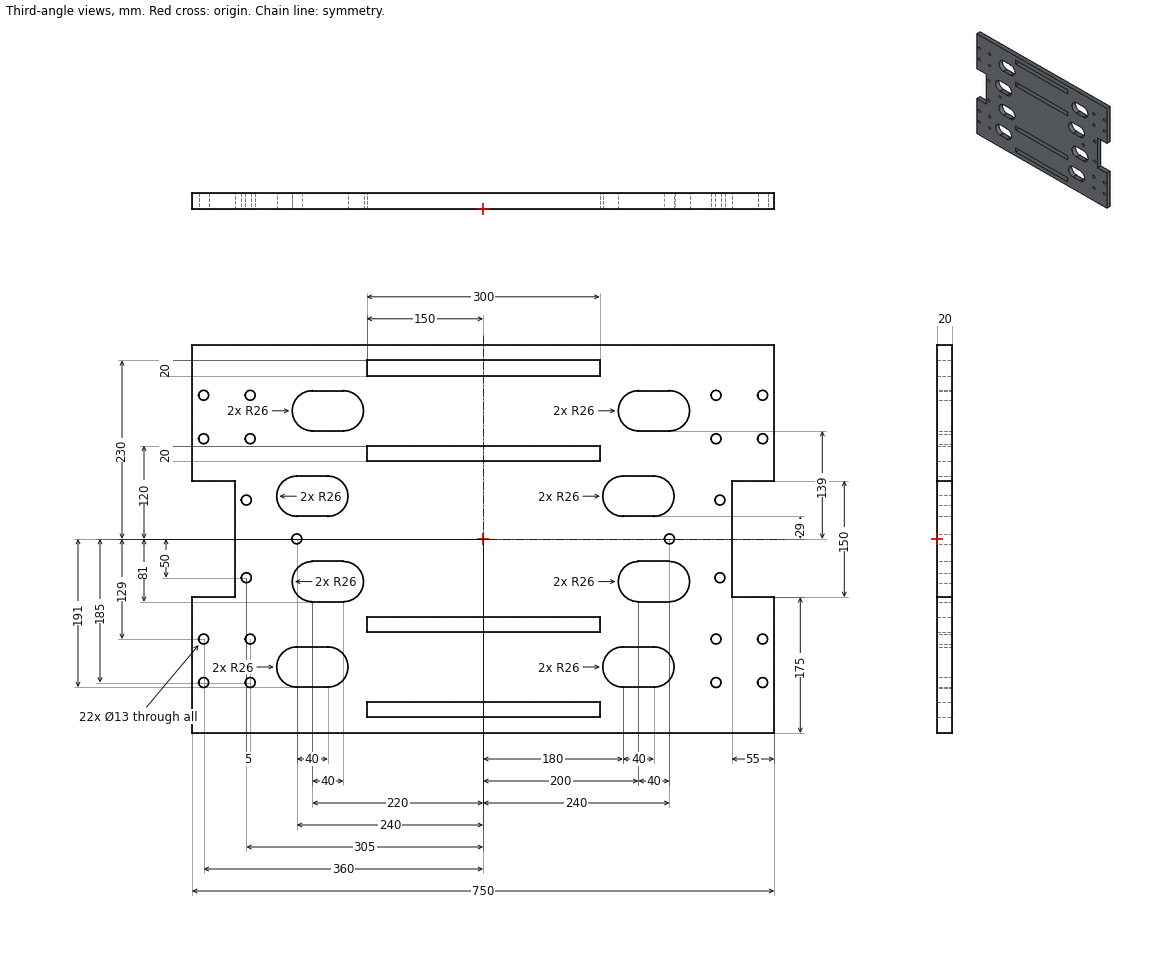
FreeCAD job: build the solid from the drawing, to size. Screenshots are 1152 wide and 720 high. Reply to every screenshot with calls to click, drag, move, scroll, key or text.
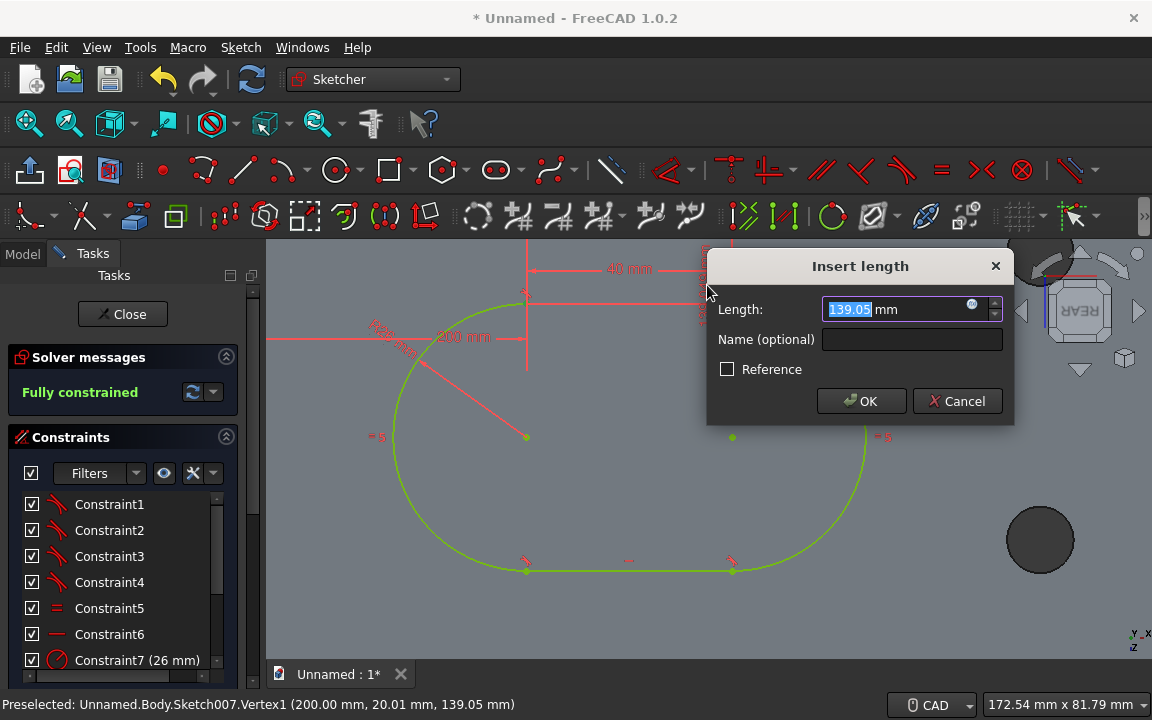
text(139)
key(Return)
key(Escape)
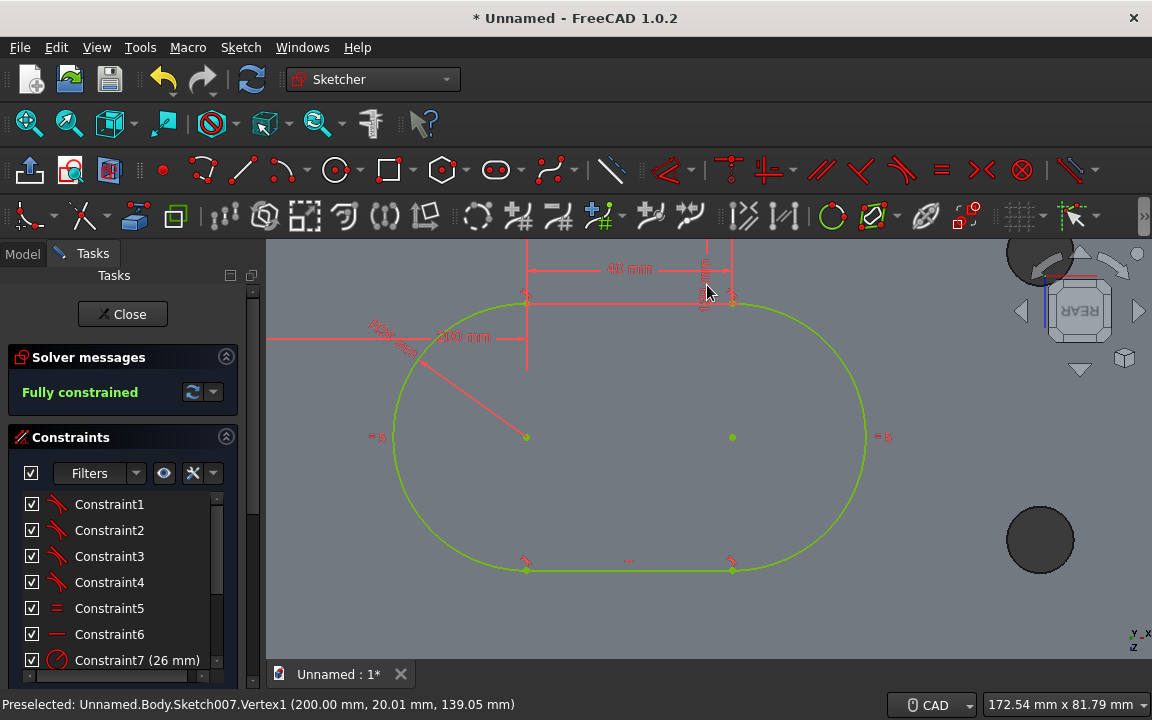
click(123, 314)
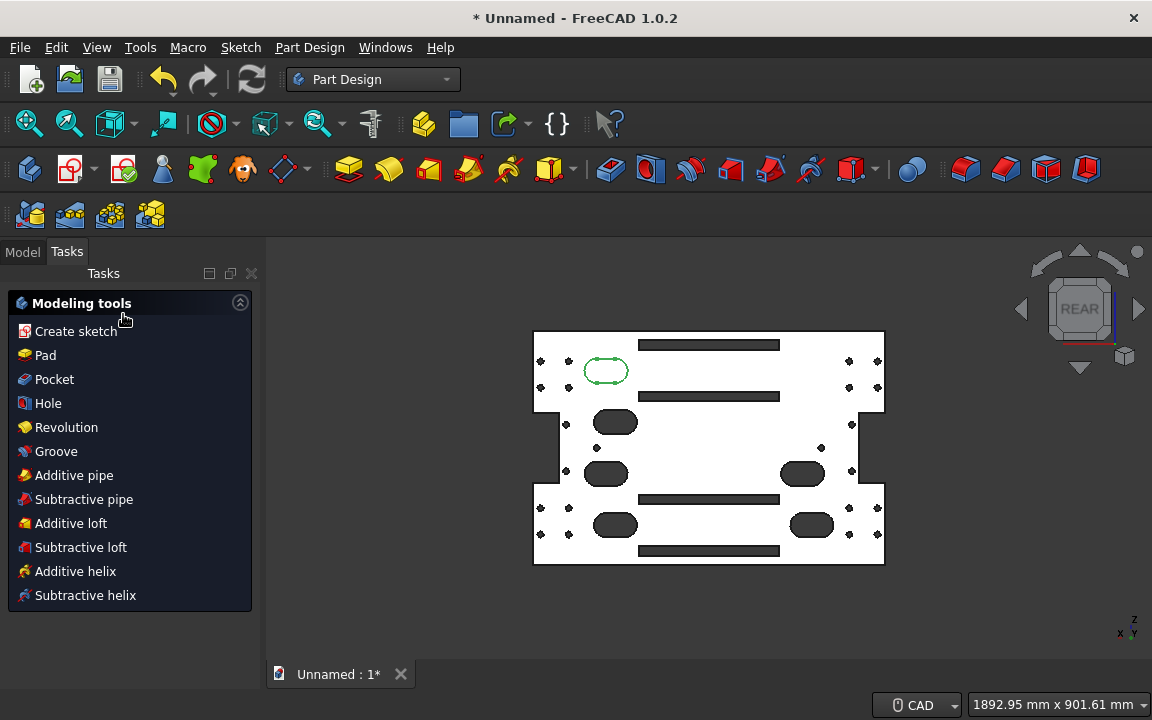
click(612, 170)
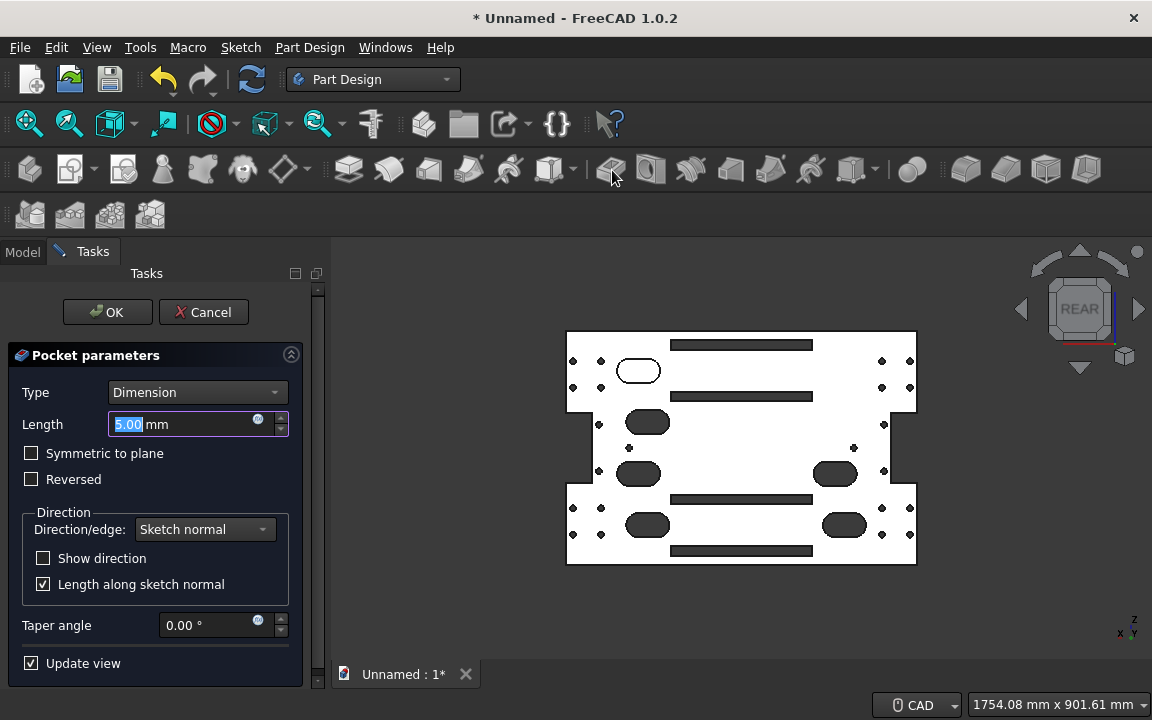
click(198, 392)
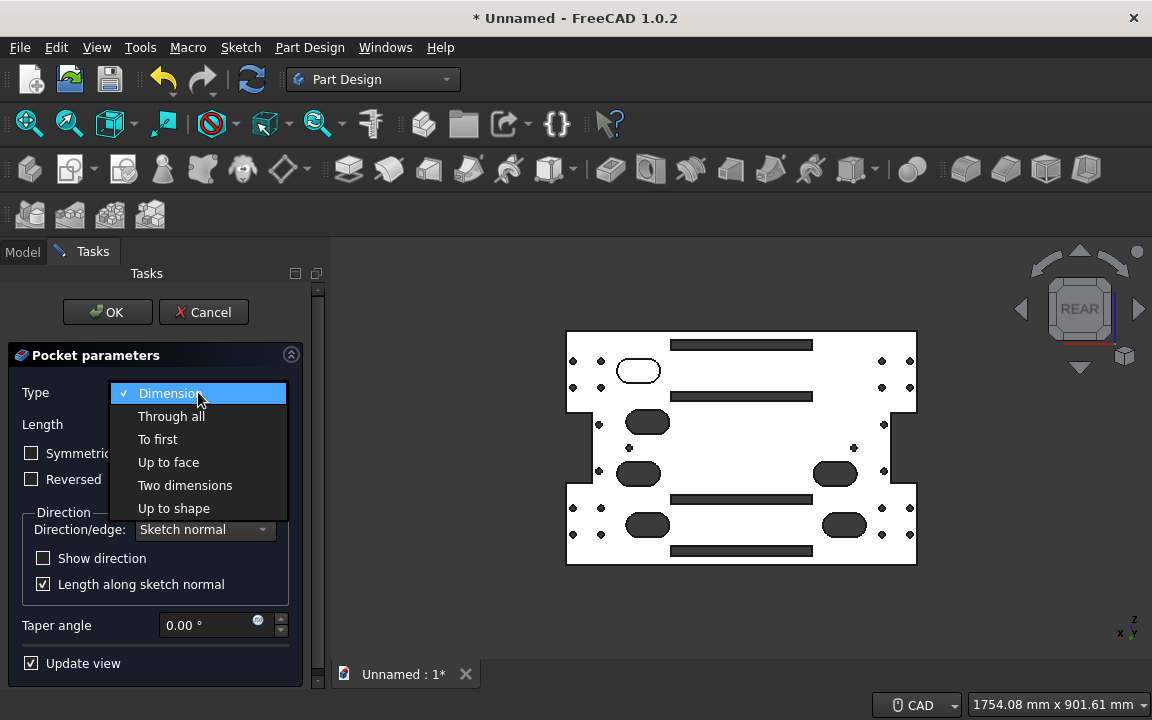
click(198, 440)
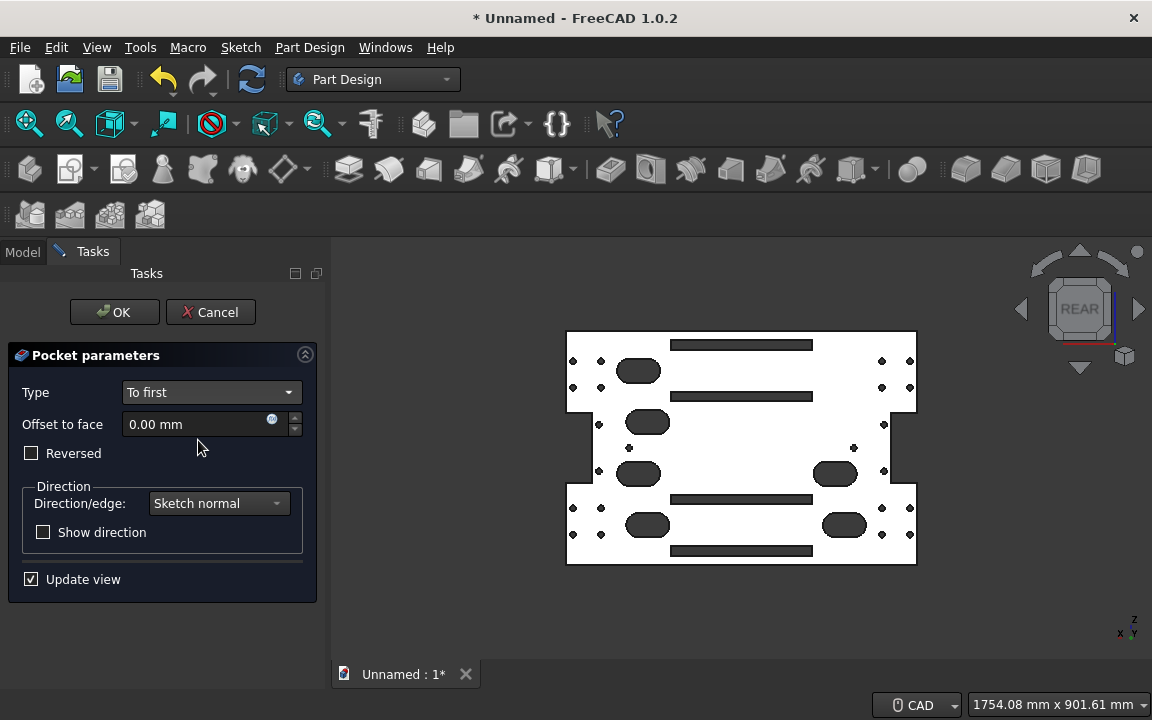
click(115, 312)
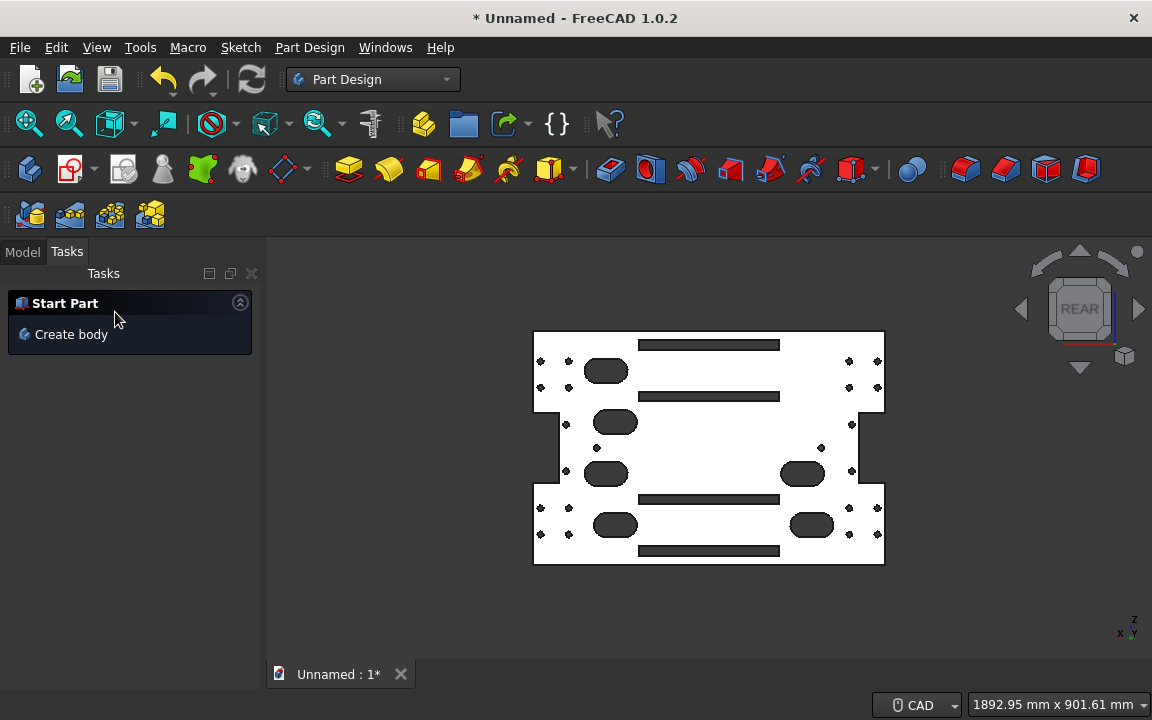
click(709, 447)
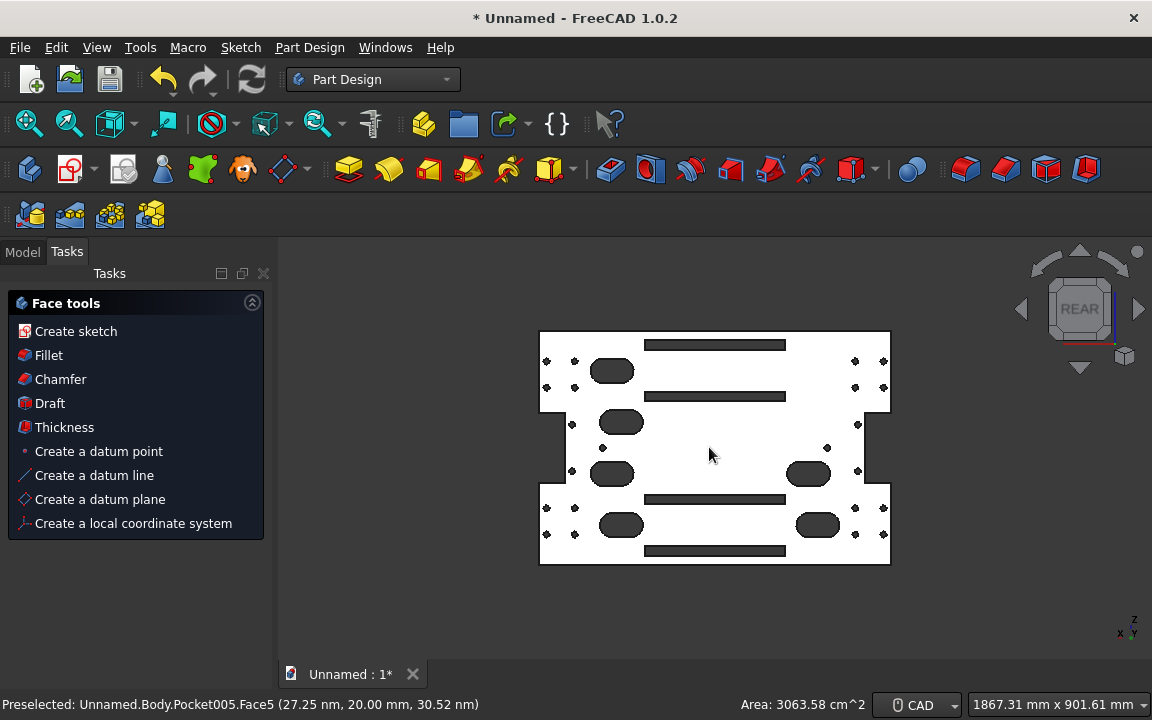
click(70, 170)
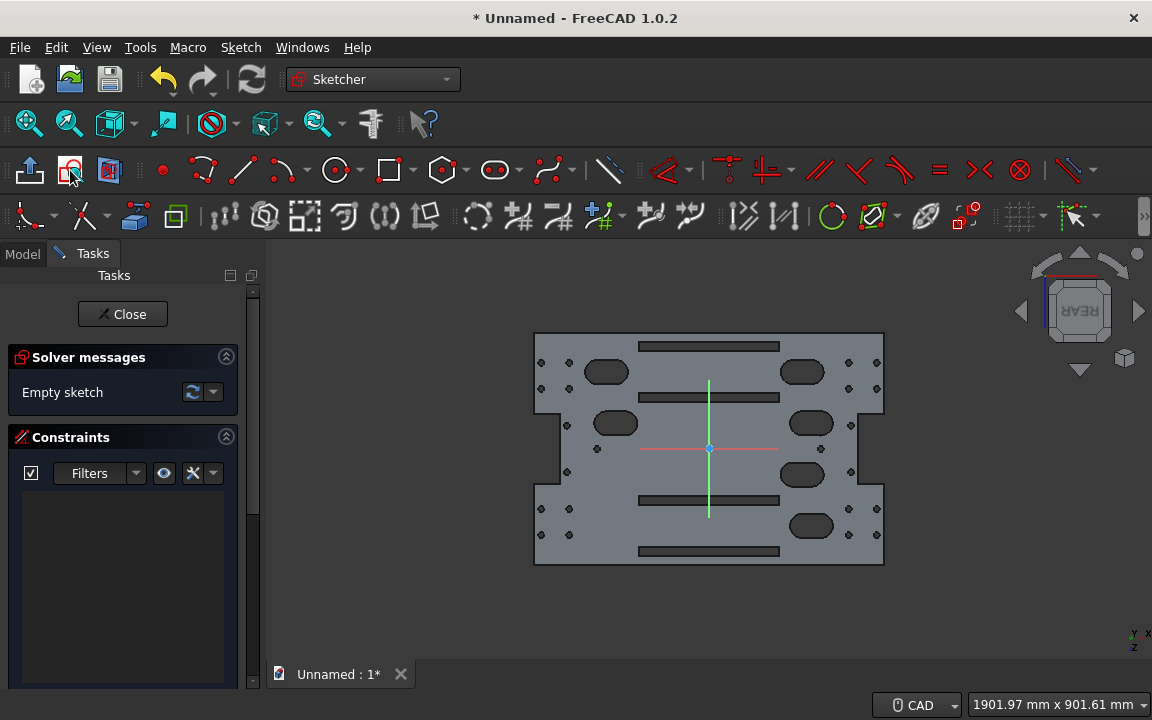
scroll(603, 477, up, 12)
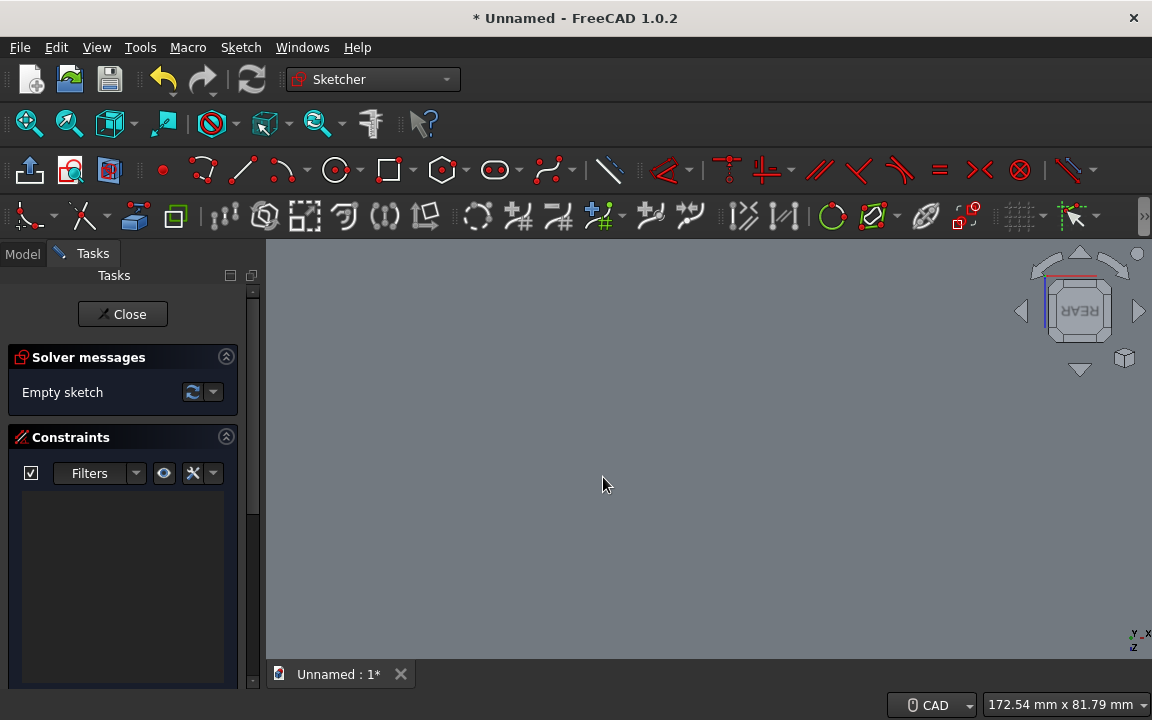
click(496, 170)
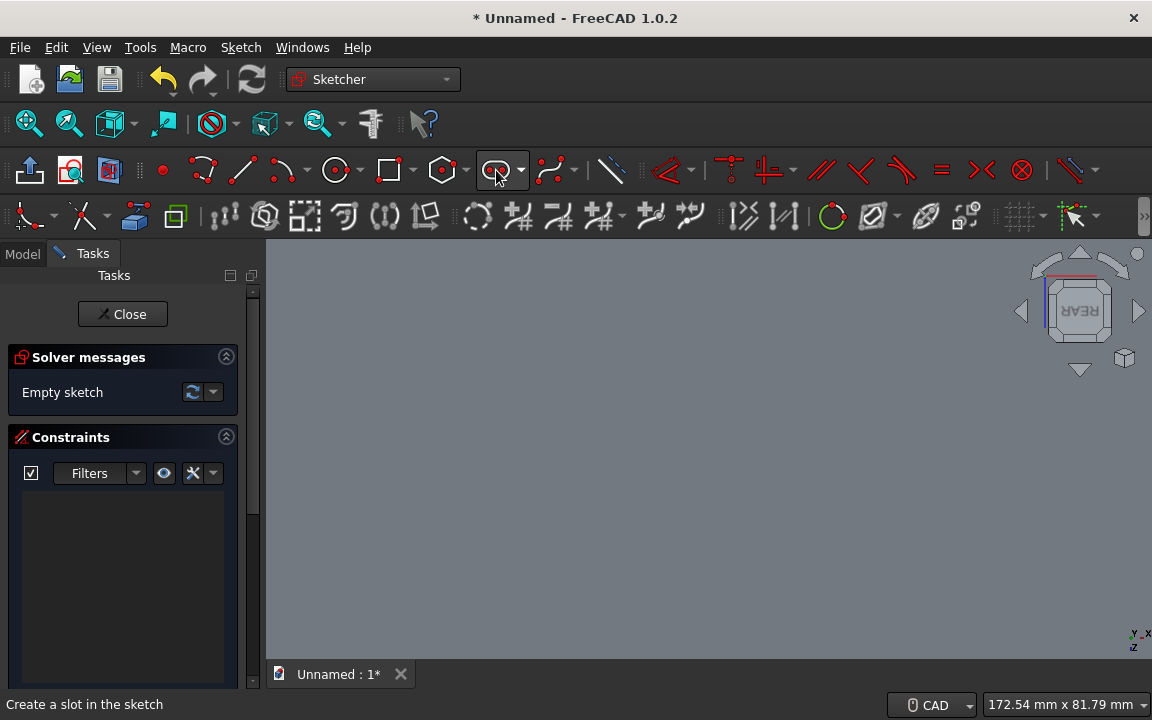
click(535, 445)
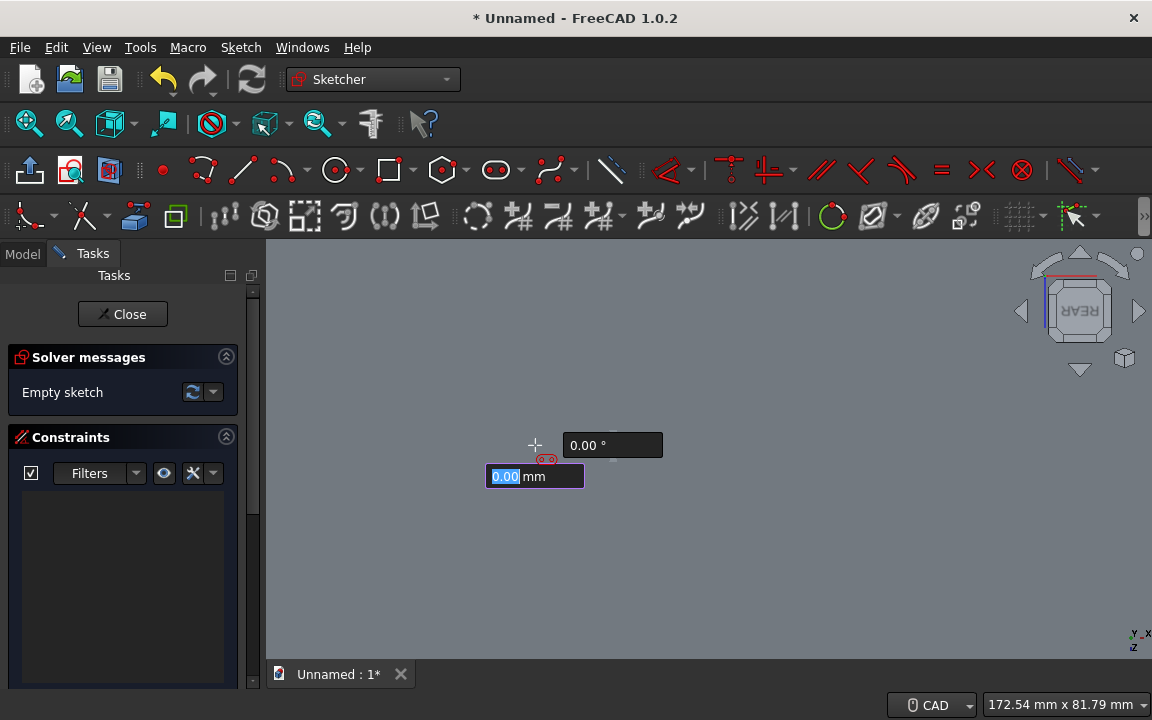
click(741, 445)